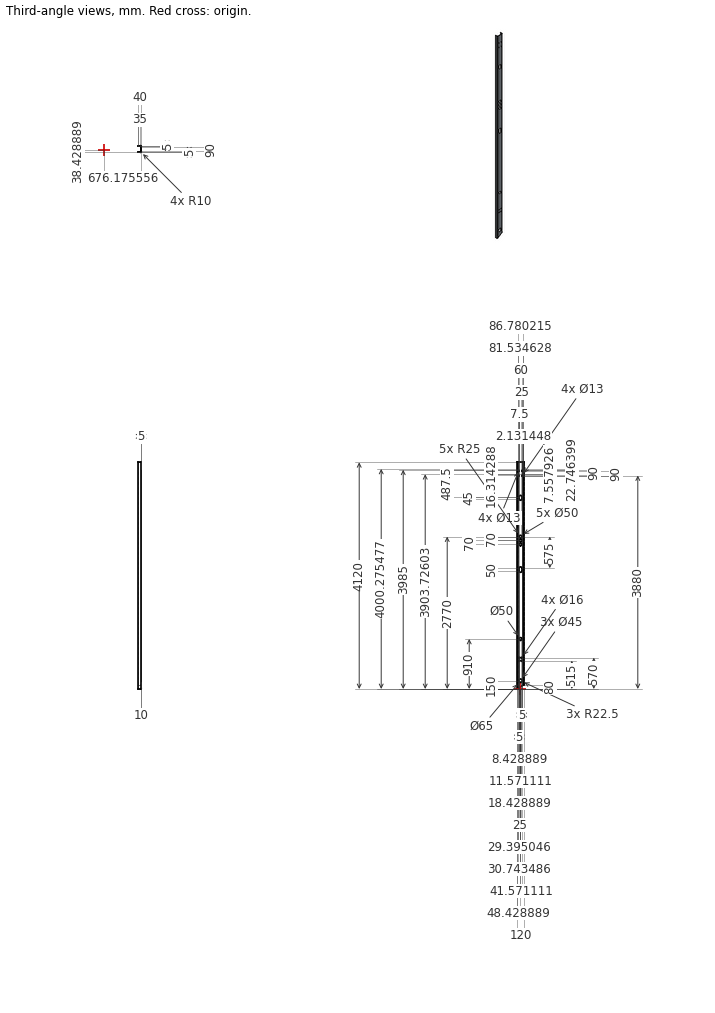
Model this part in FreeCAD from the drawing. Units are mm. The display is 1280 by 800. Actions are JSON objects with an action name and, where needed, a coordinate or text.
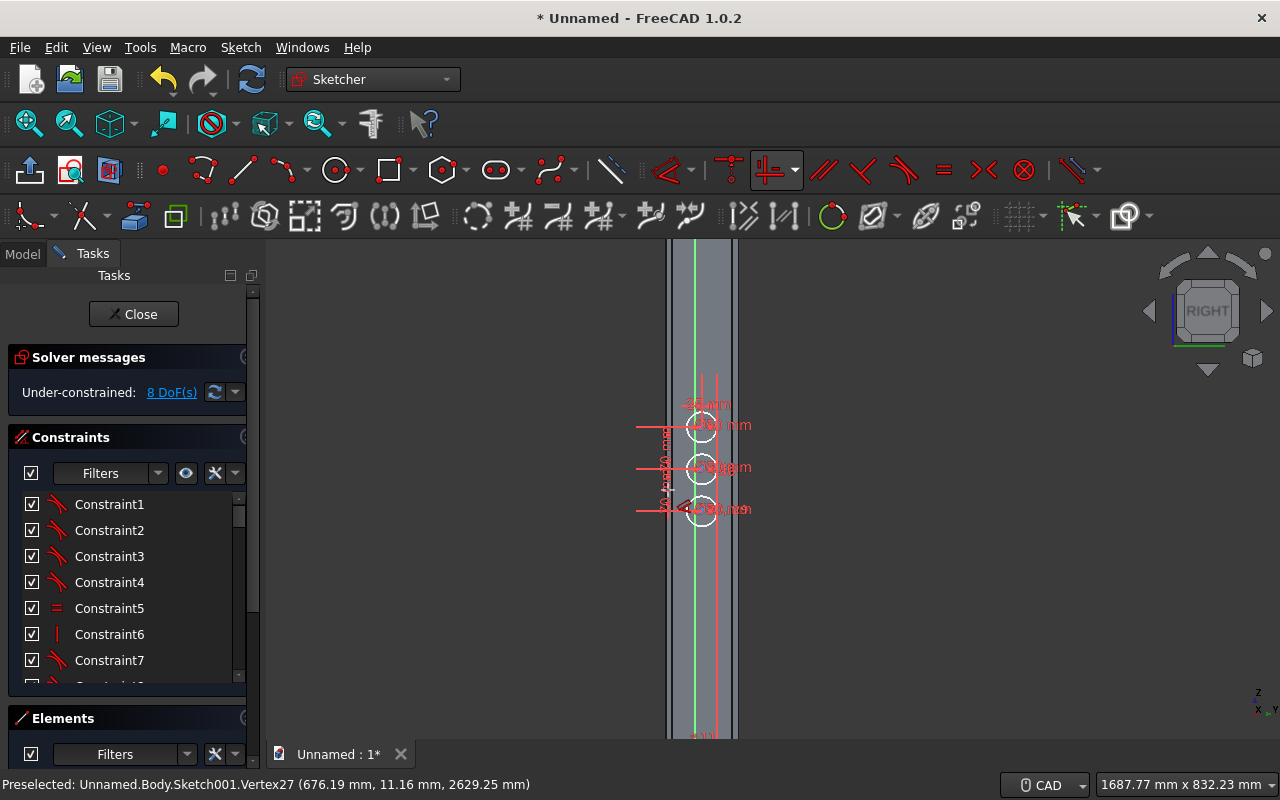
{"action": "scroll", "coordinate": [705, 426], "scroll_direction": "down", "scroll_amount": 10}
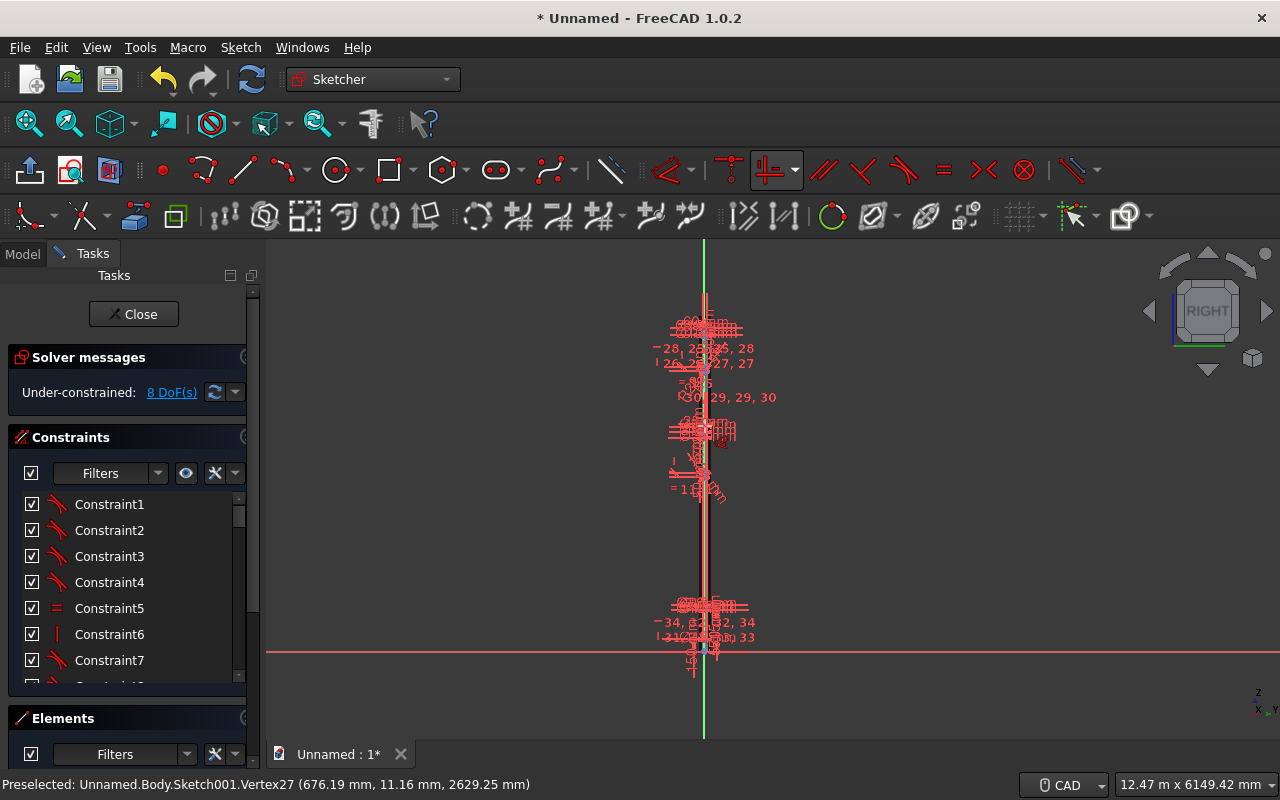
{"action": "scroll", "coordinate": [703, 477], "scroll_direction": "up", "scroll_amount": 15}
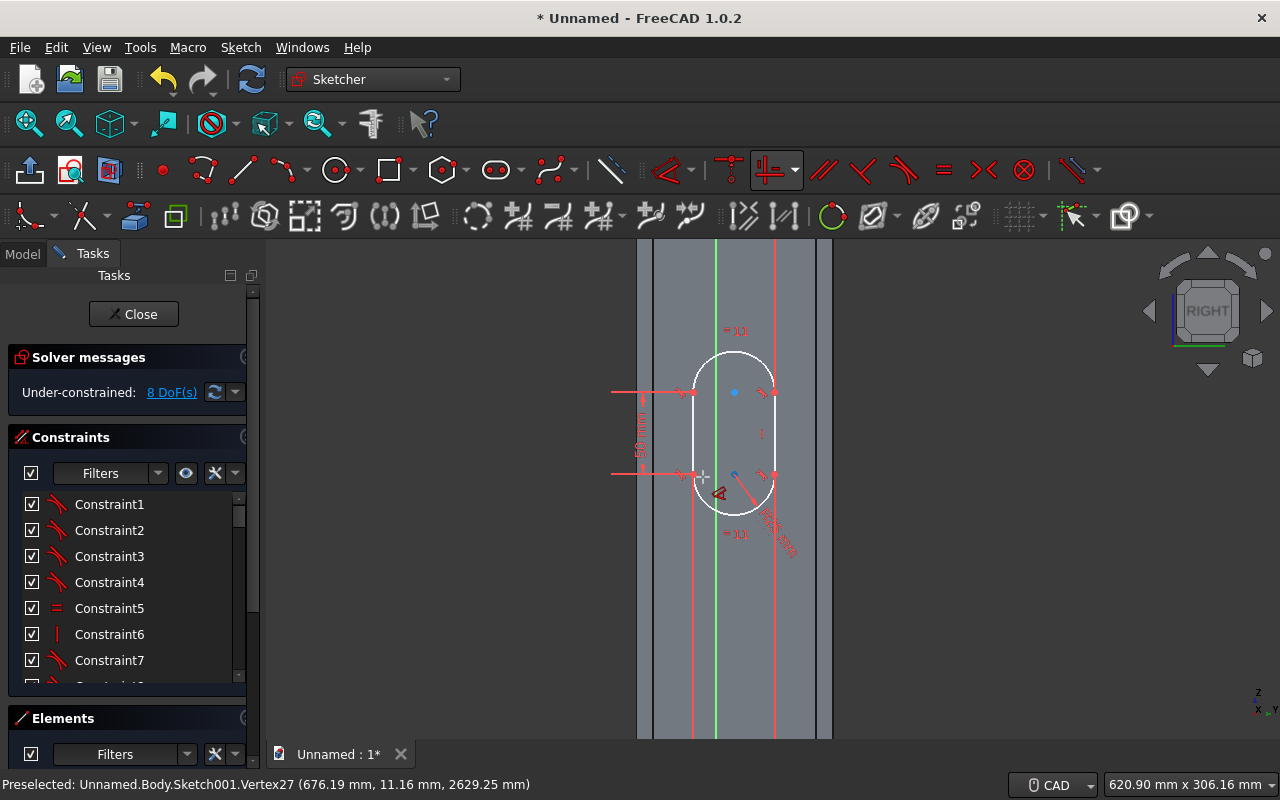
{"action": "left_click", "coordinate": [693, 474]}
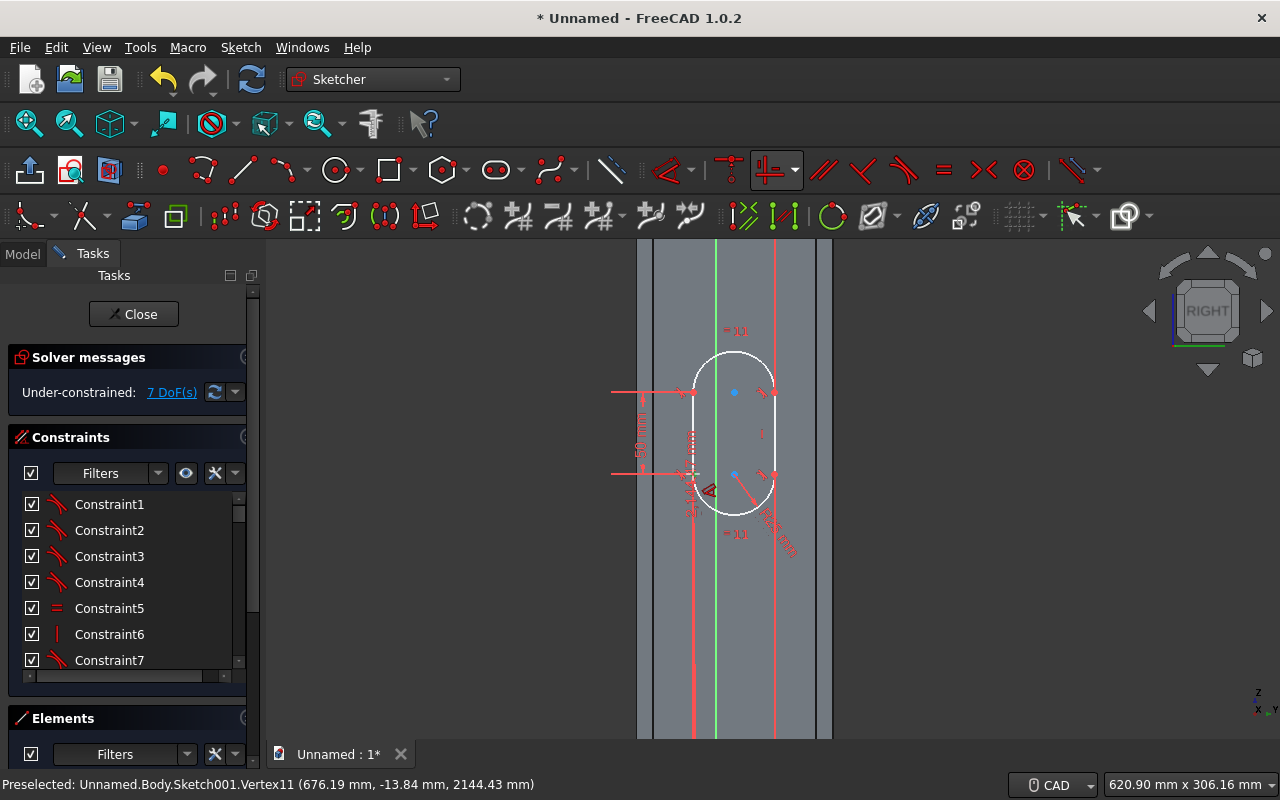
{"action": "scroll", "coordinate": [703, 477], "scroll_direction": "down", "scroll_amount": 15}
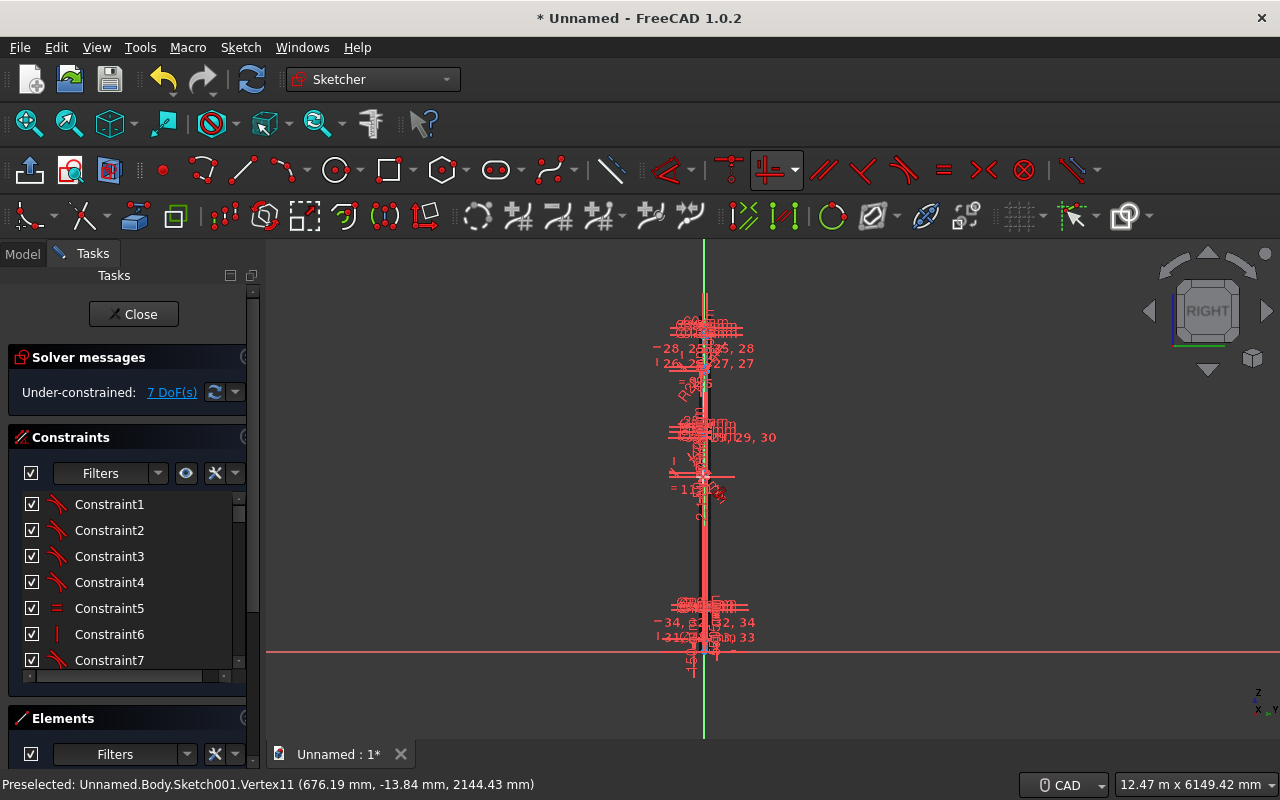
{"action": "scroll", "coordinate": [705, 639], "scroll_direction": "up", "scroll_amount": 15}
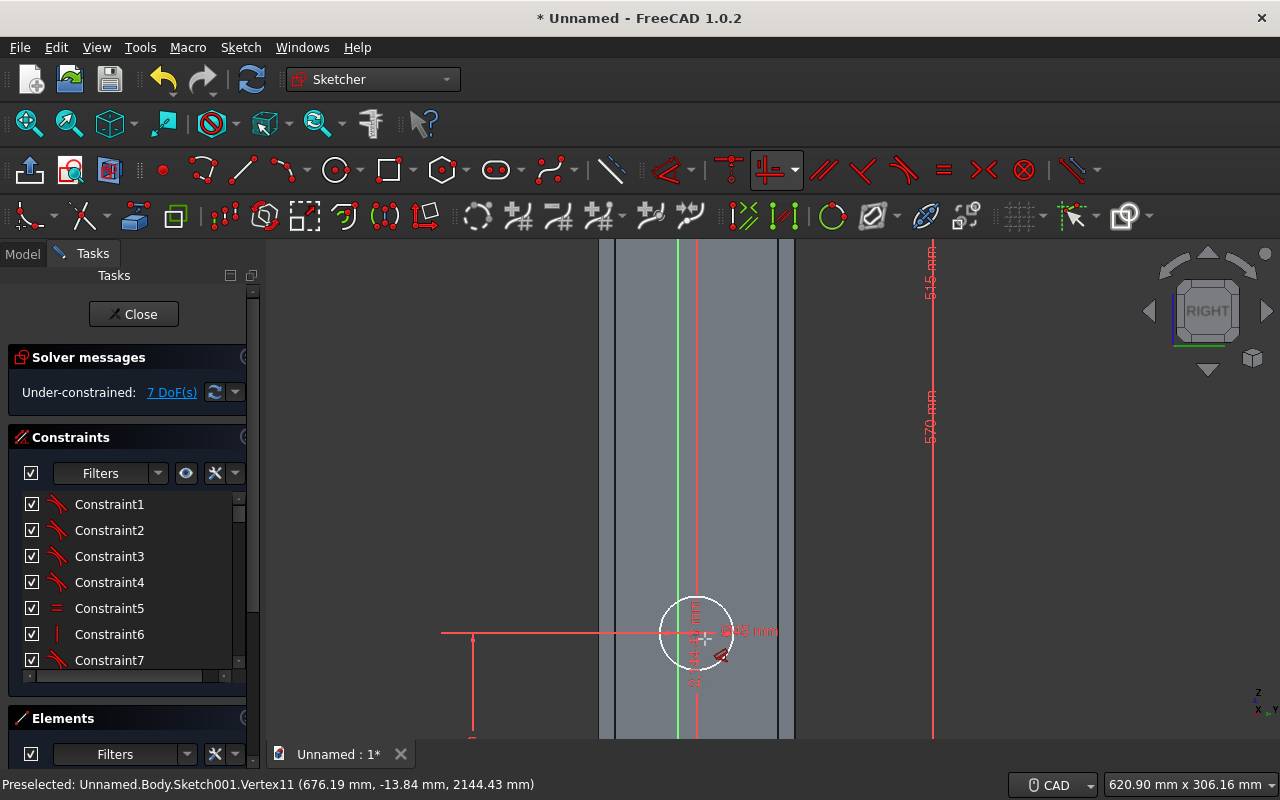
{"action": "left_click", "coordinate": [697, 633]}
{"action": "left_click", "coordinate": [661, 691]}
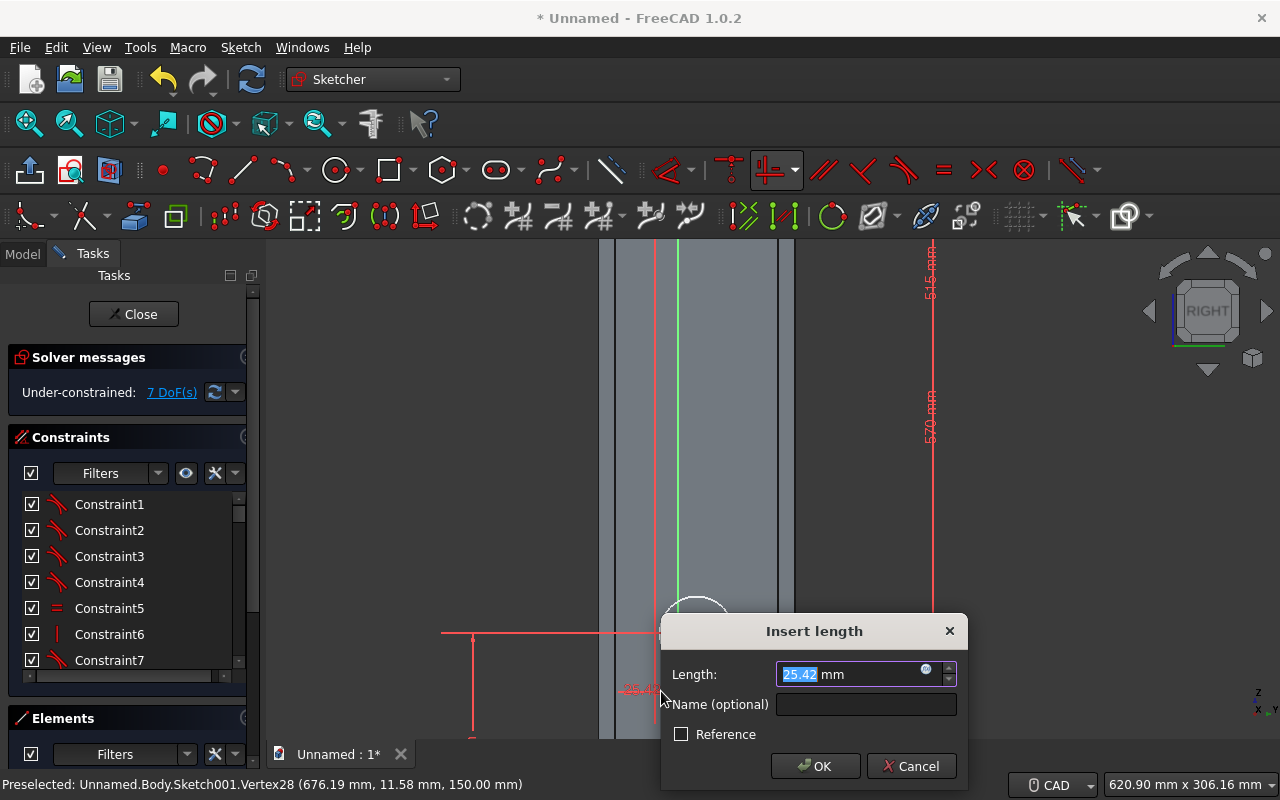
{"action": "type", "text": "25"}
{"action": "key", "text": "Return"}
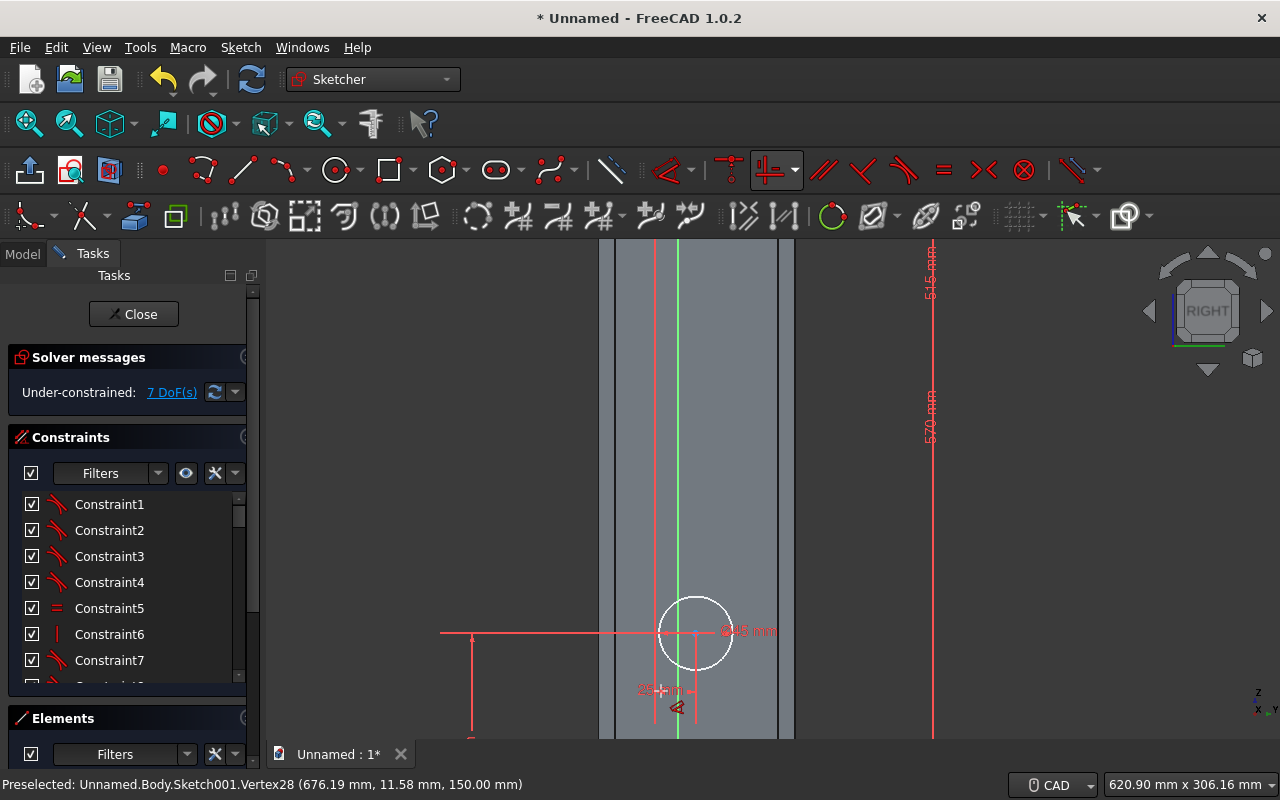
{"action": "scroll", "coordinate": [705, 639], "scroll_direction": "down", "scroll_amount": 15}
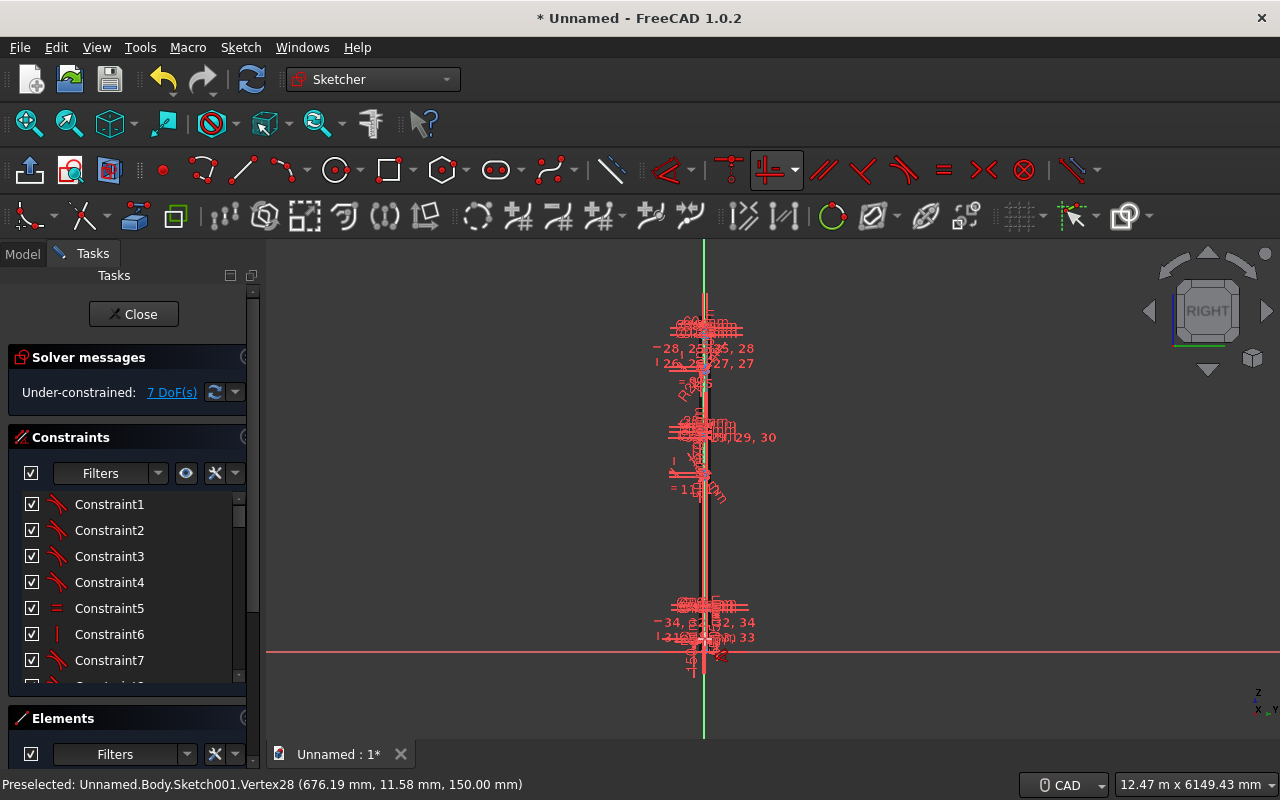
{"action": "scroll", "coordinate": [703, 328], "scroll_direction": "up", "scroll_amount": 5}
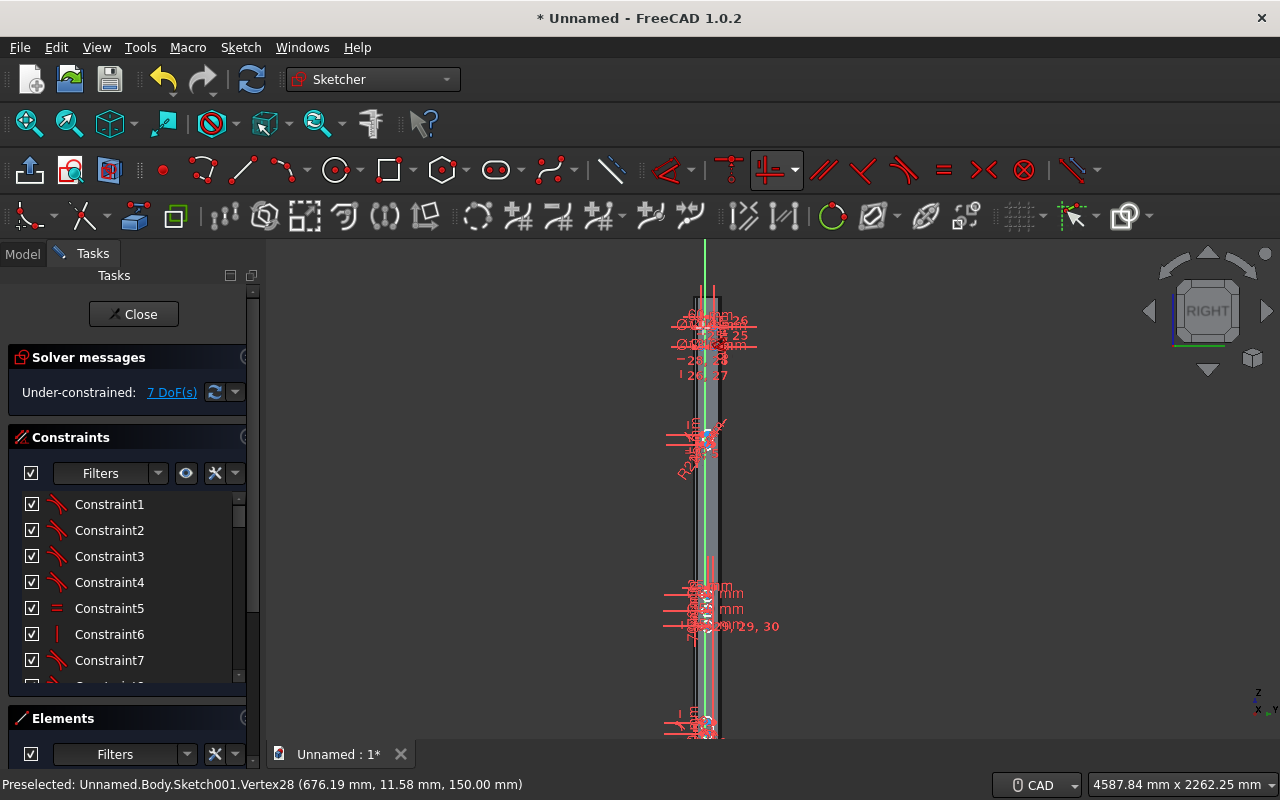
{"action": "left_click", "coordinate": [701, 327]}
{"action": "left_click", "coordinate": [667, 519]}